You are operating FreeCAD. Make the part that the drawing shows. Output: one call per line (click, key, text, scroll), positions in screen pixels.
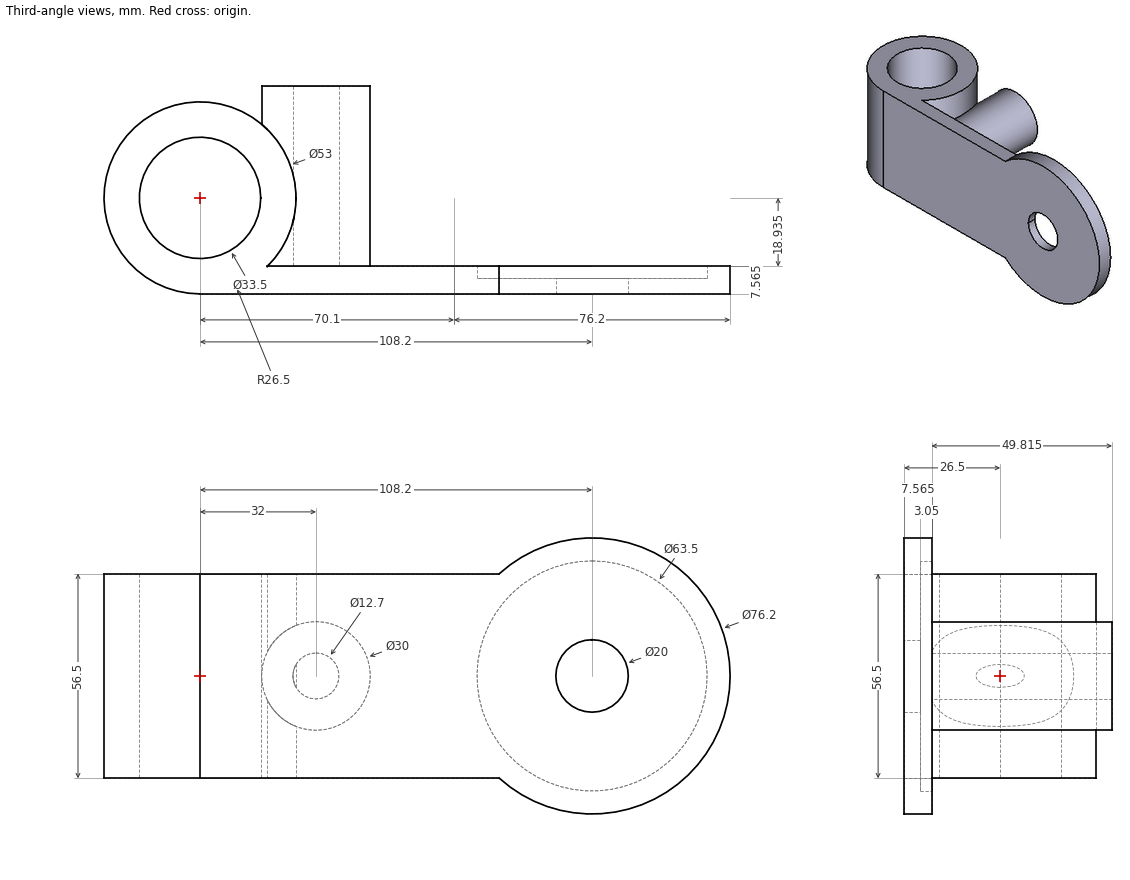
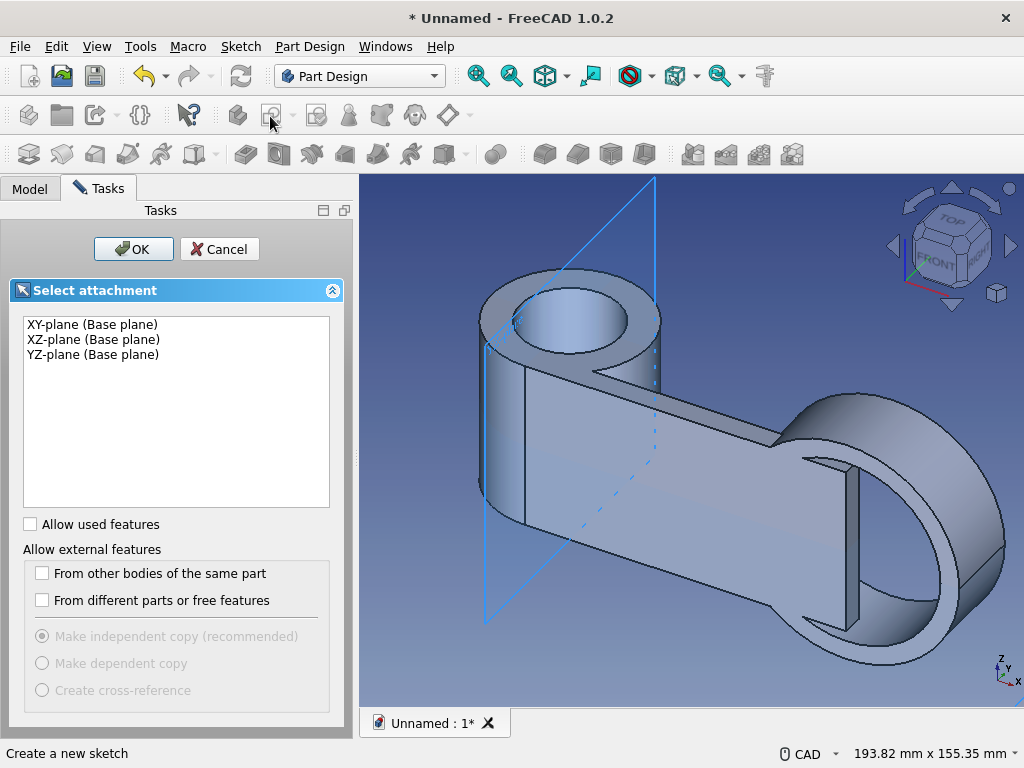
click(84, 324)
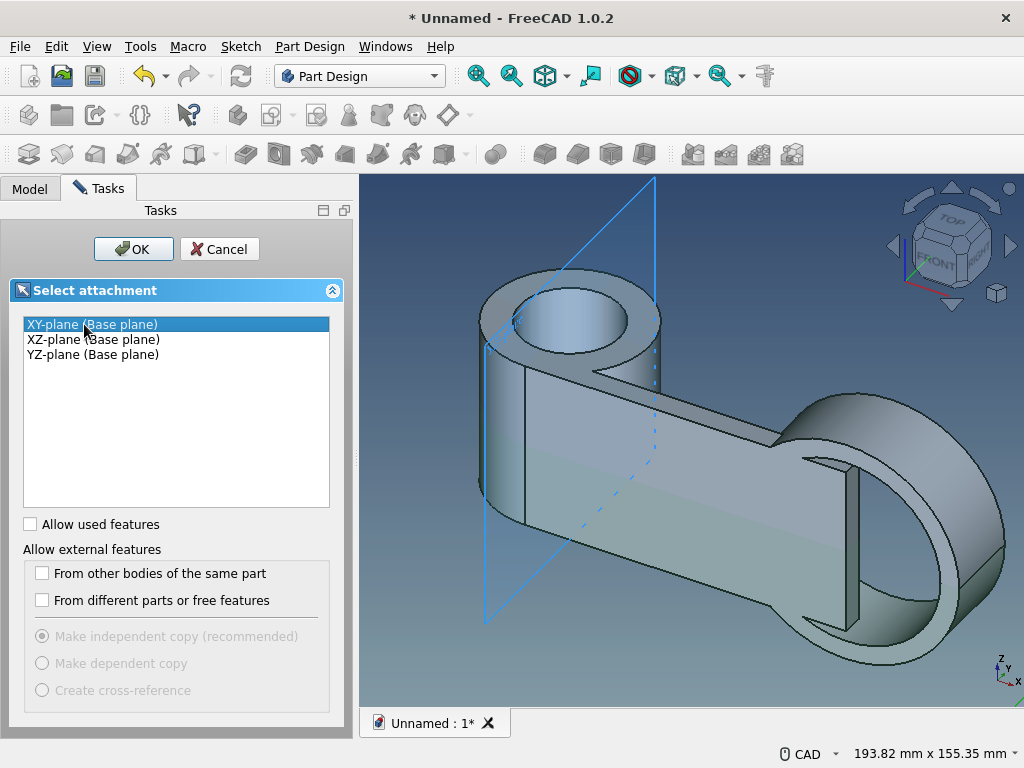
click(134, 249)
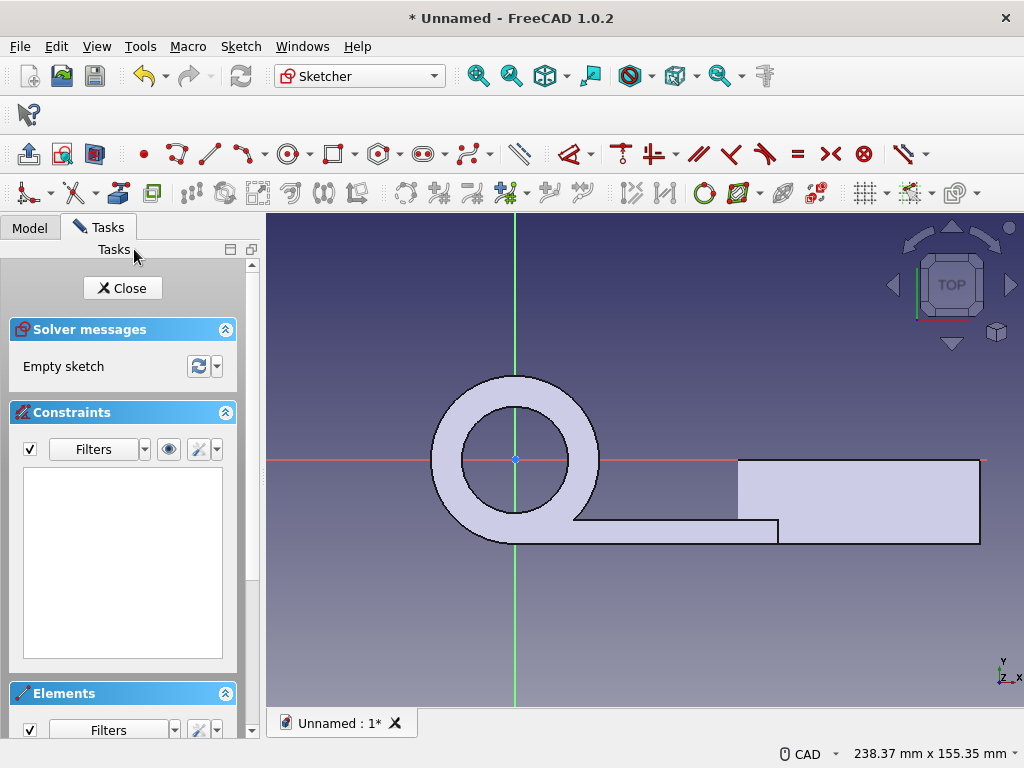
key(q)
key(s)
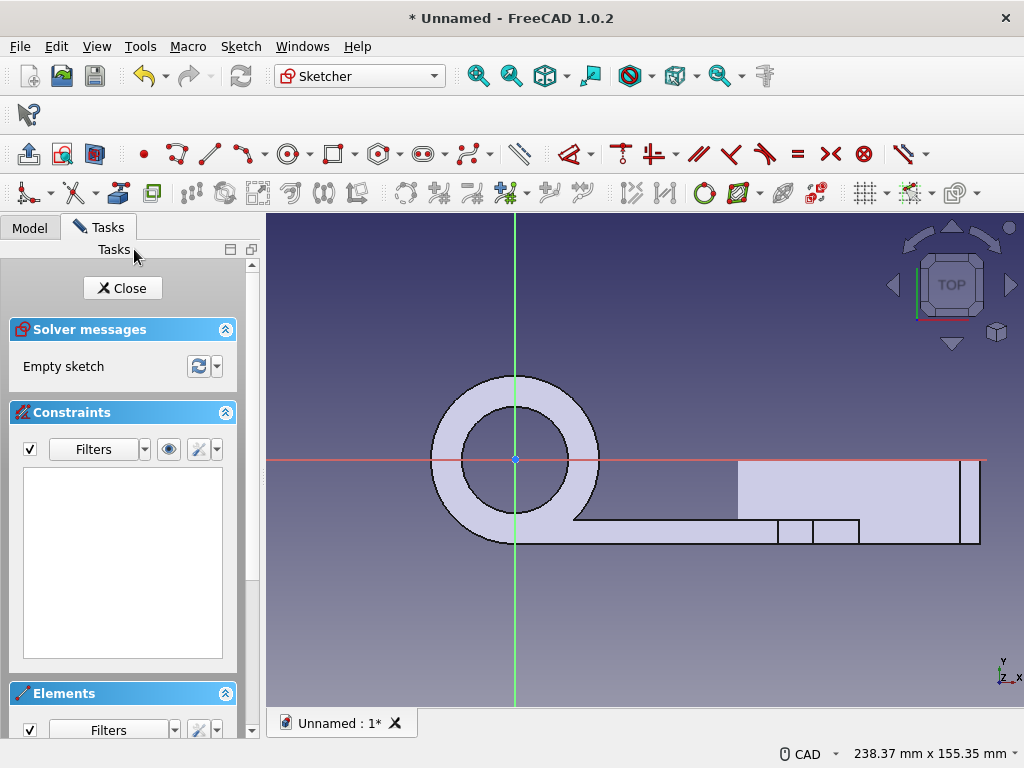
scroll(294, 399, down, 2)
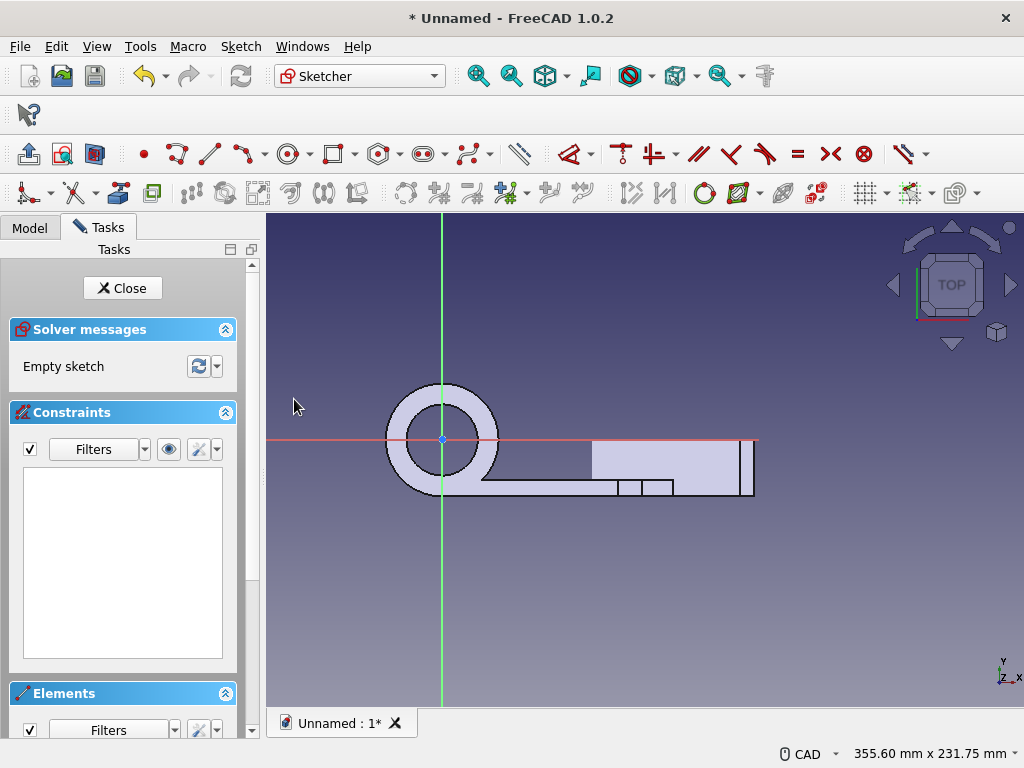
key(g)
key(r)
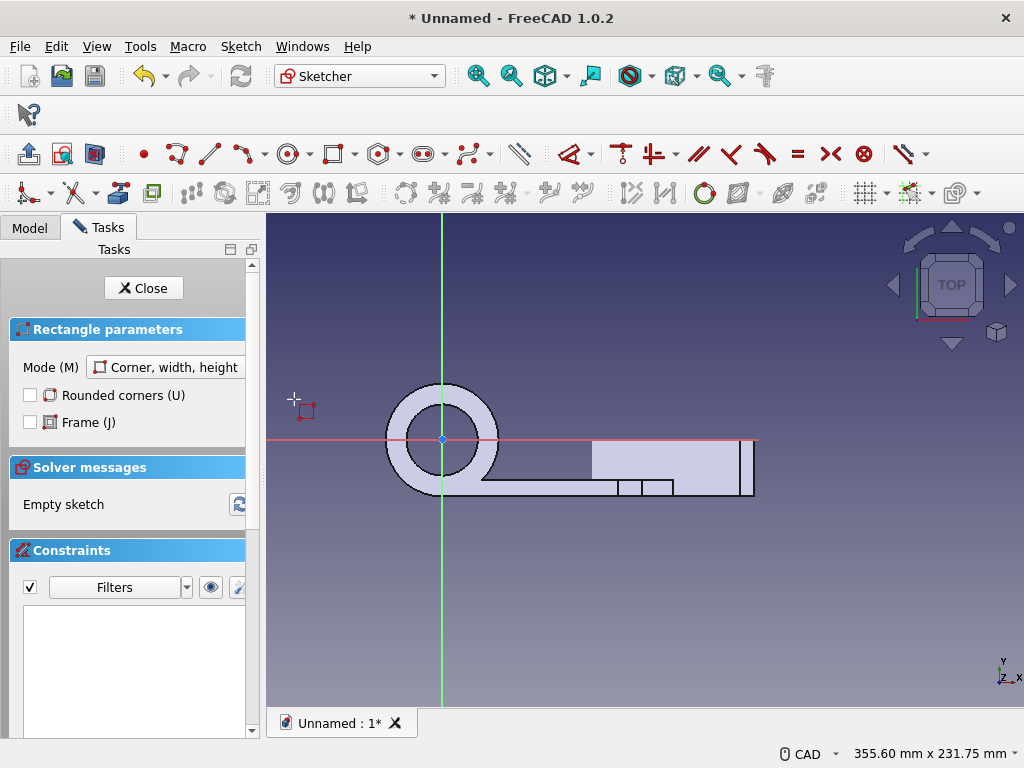
click(592, 440)
move(754, 480)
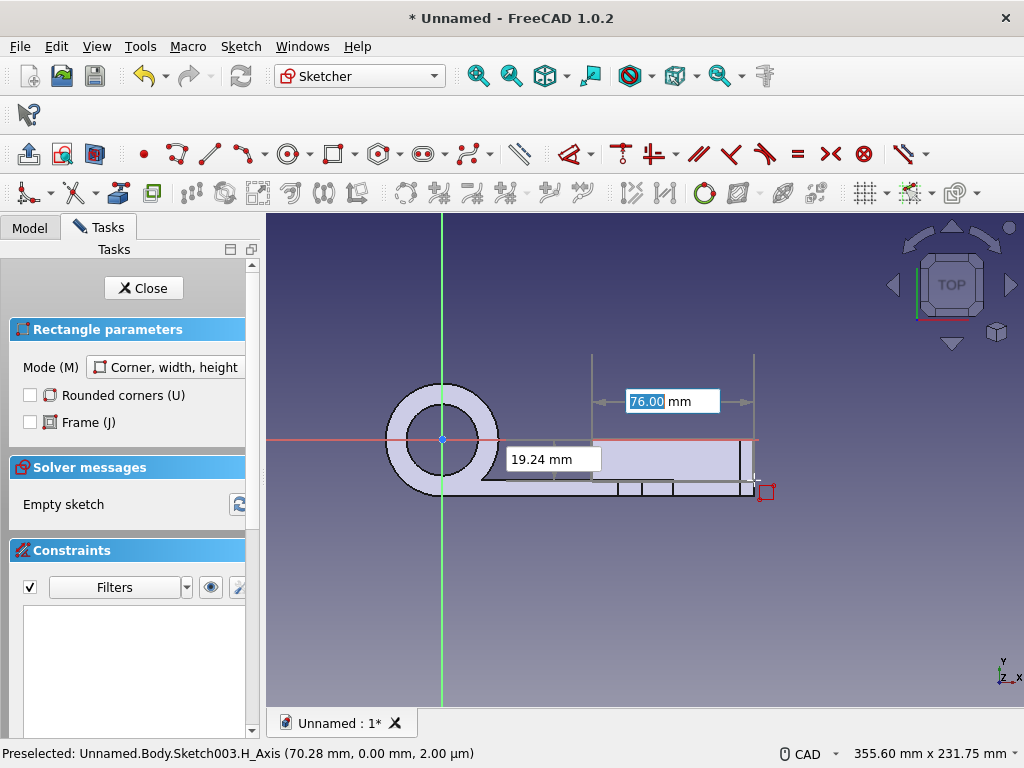
text(76.2)
key(Tab)
text(18.935)
key(Return)
key(Escape)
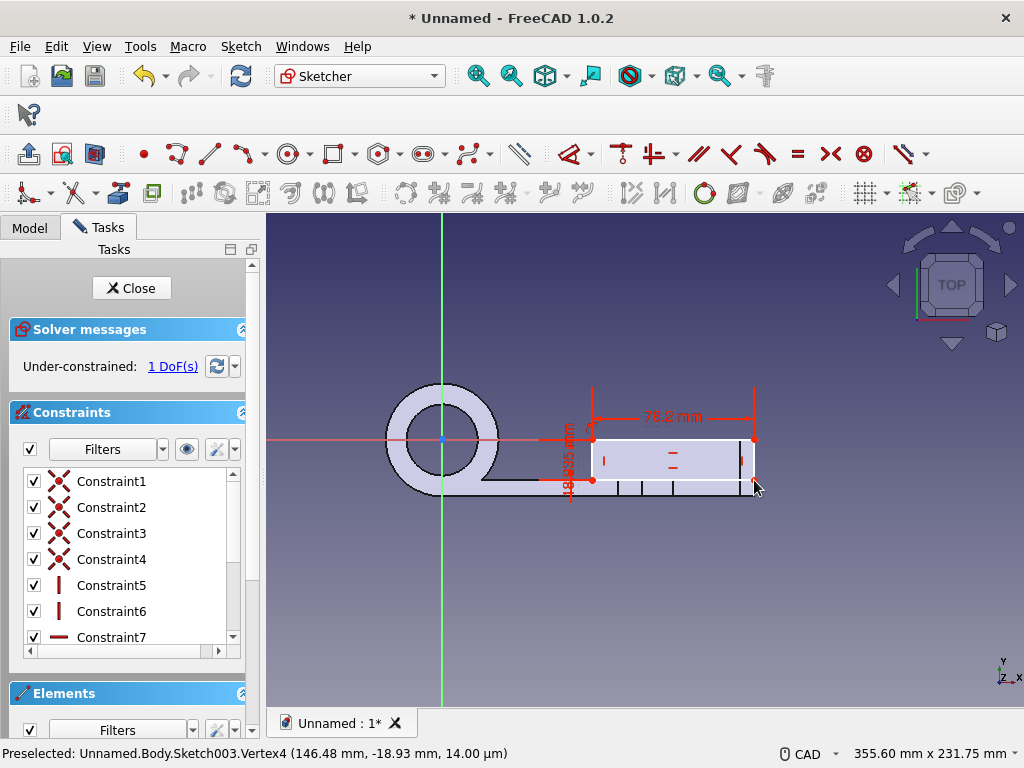
click(568, 154)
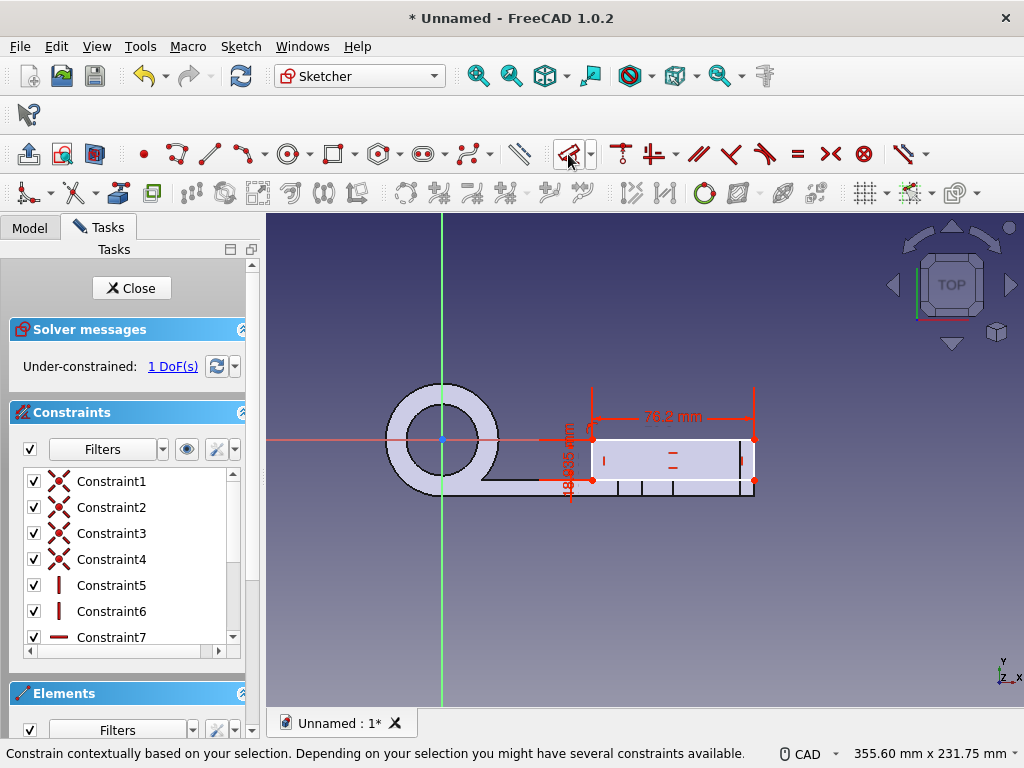
click(592, 440)
click(517, 406)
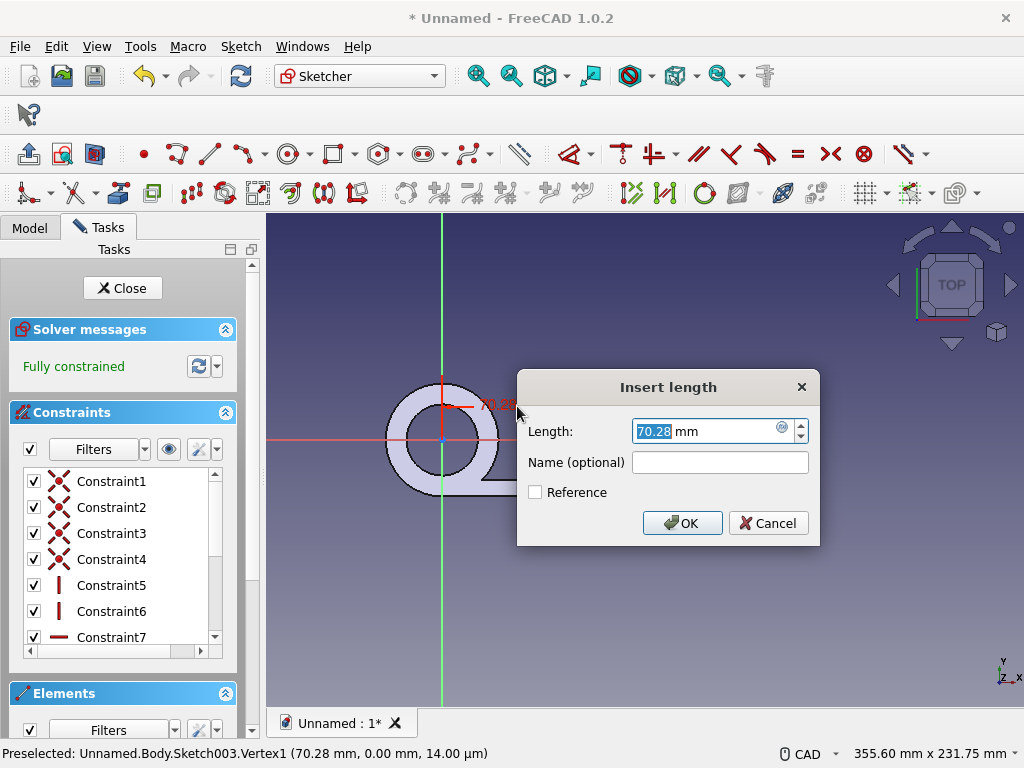
text(70.1)
key(Return)
key(Escape)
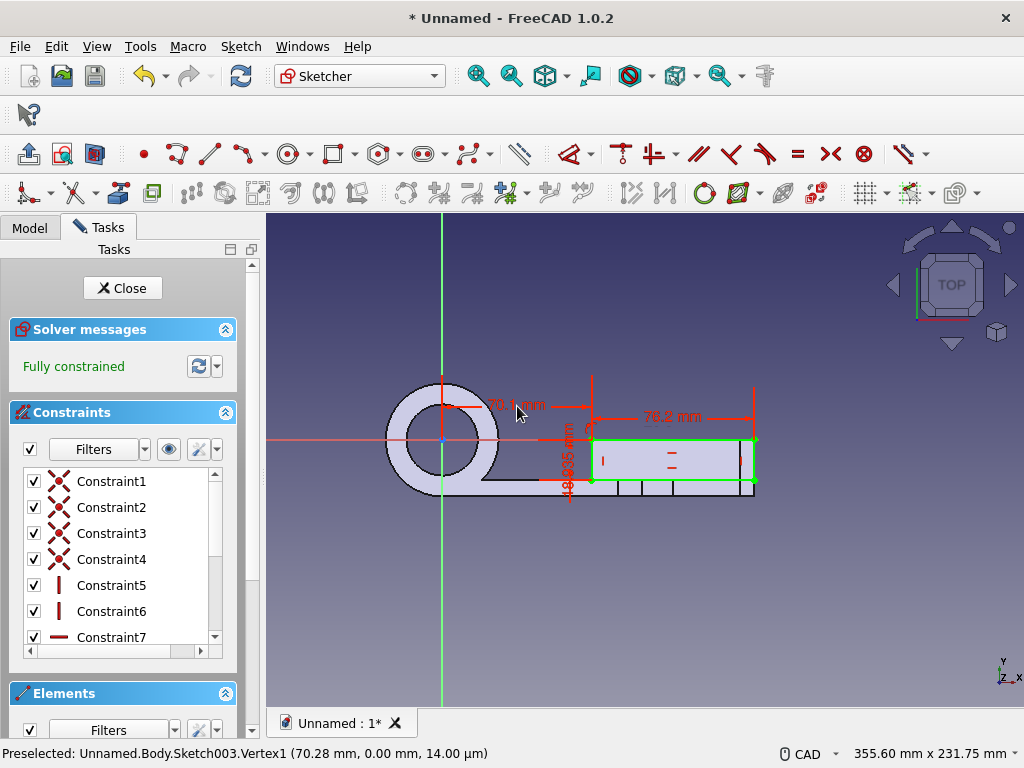
click(123, 288)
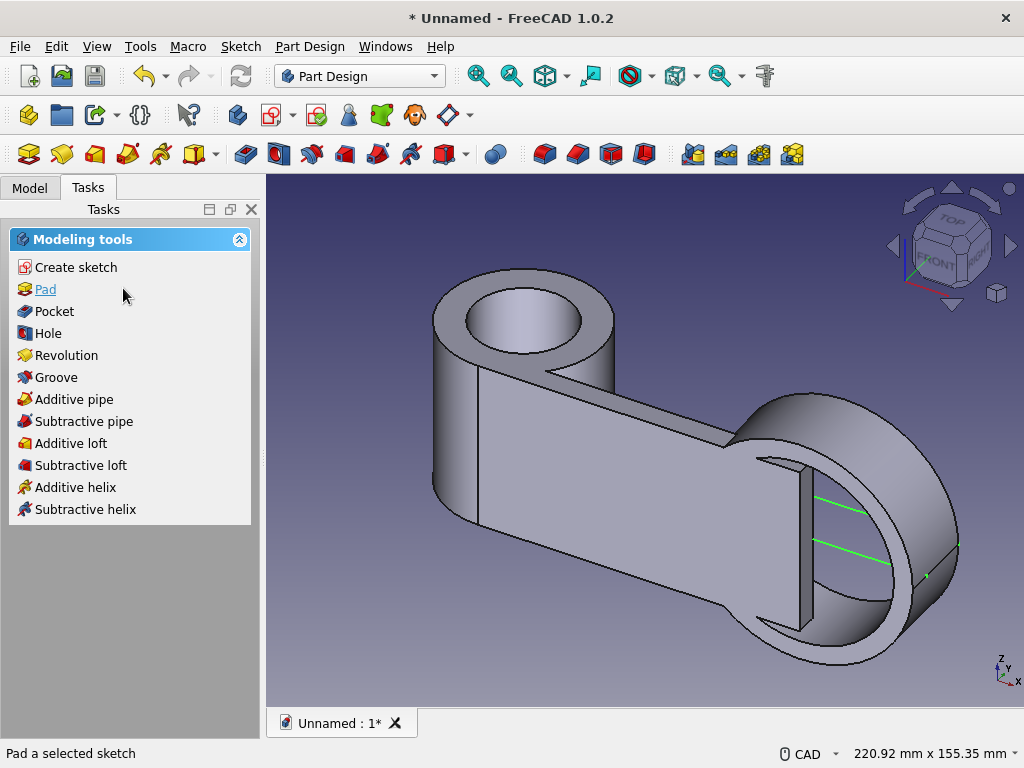
click(246, 154)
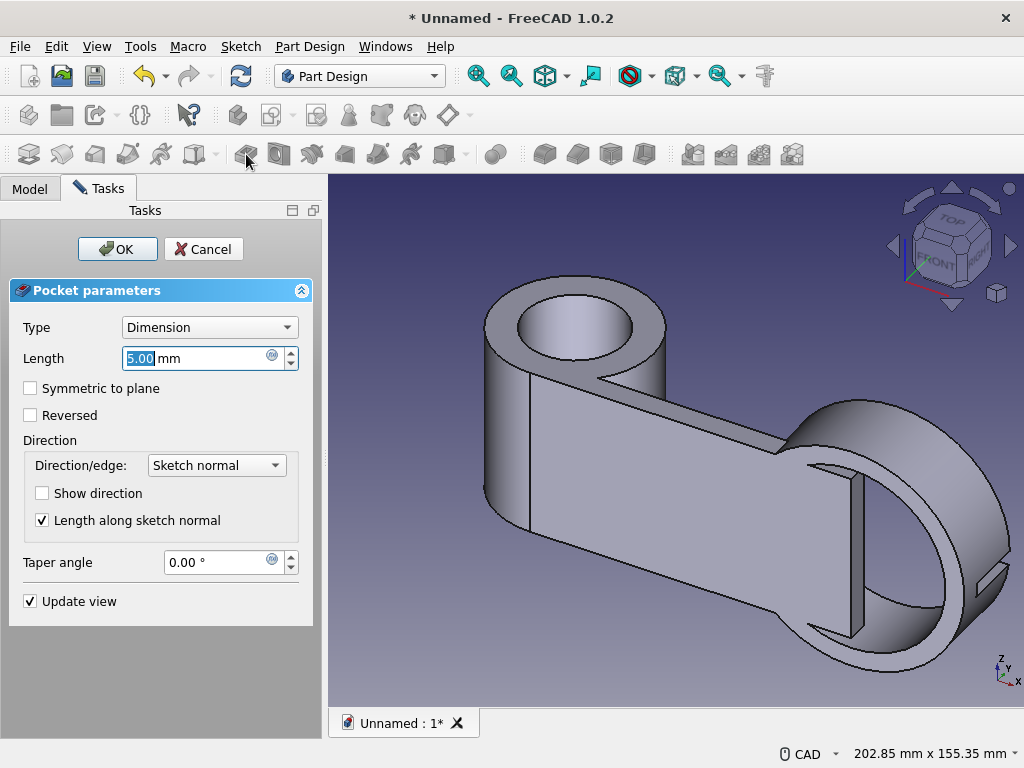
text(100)
key(Tab)